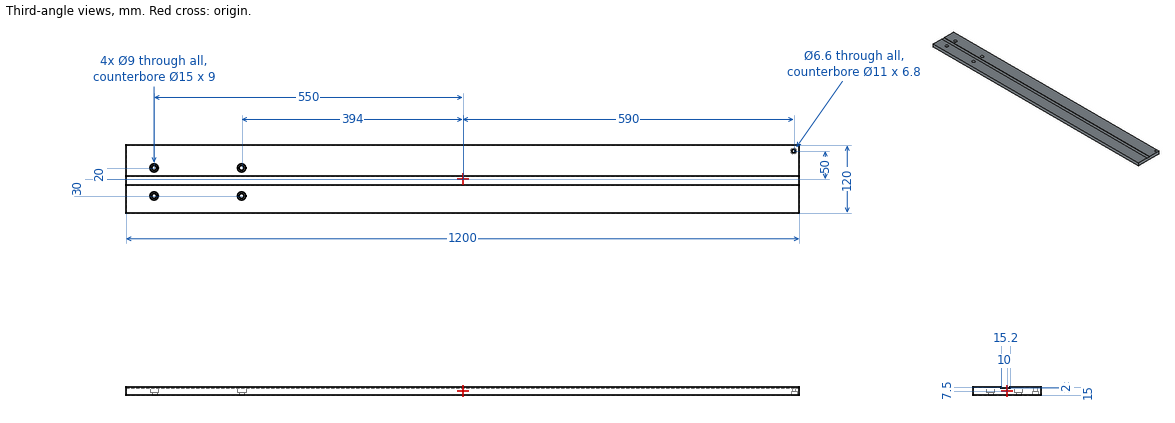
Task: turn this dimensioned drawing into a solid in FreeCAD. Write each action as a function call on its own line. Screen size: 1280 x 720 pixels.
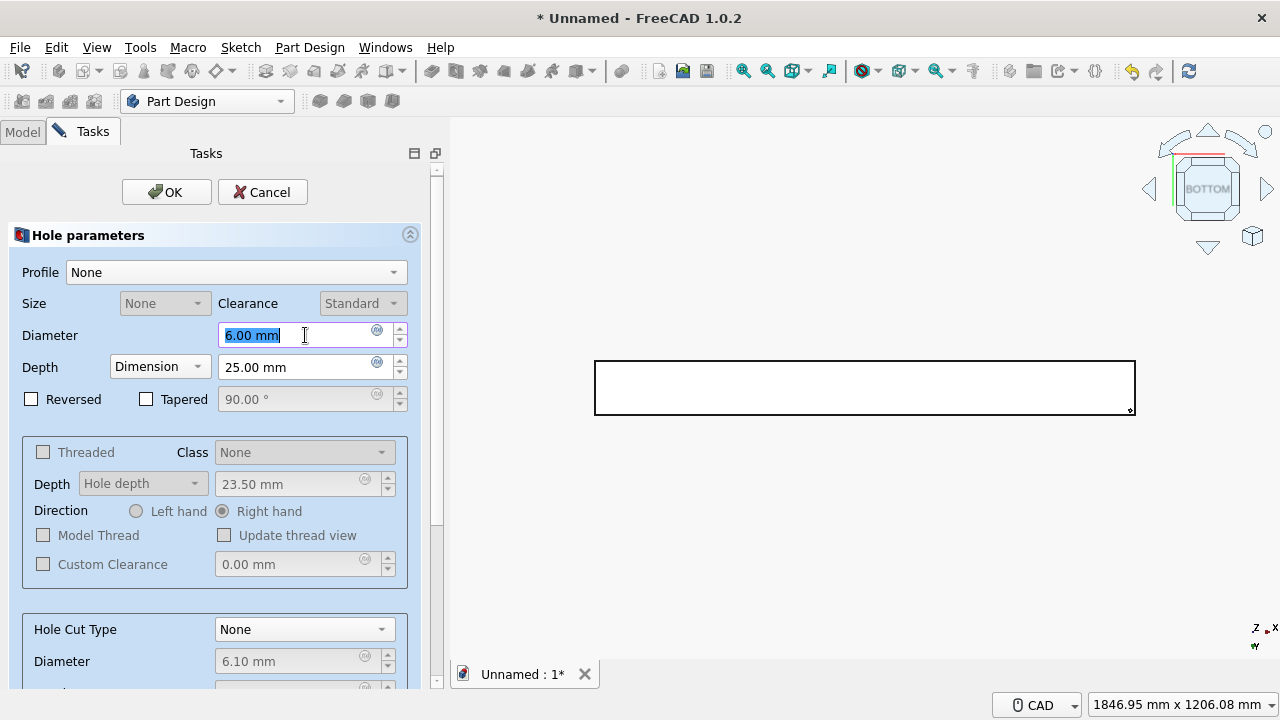
text(6.6)
key(Tab)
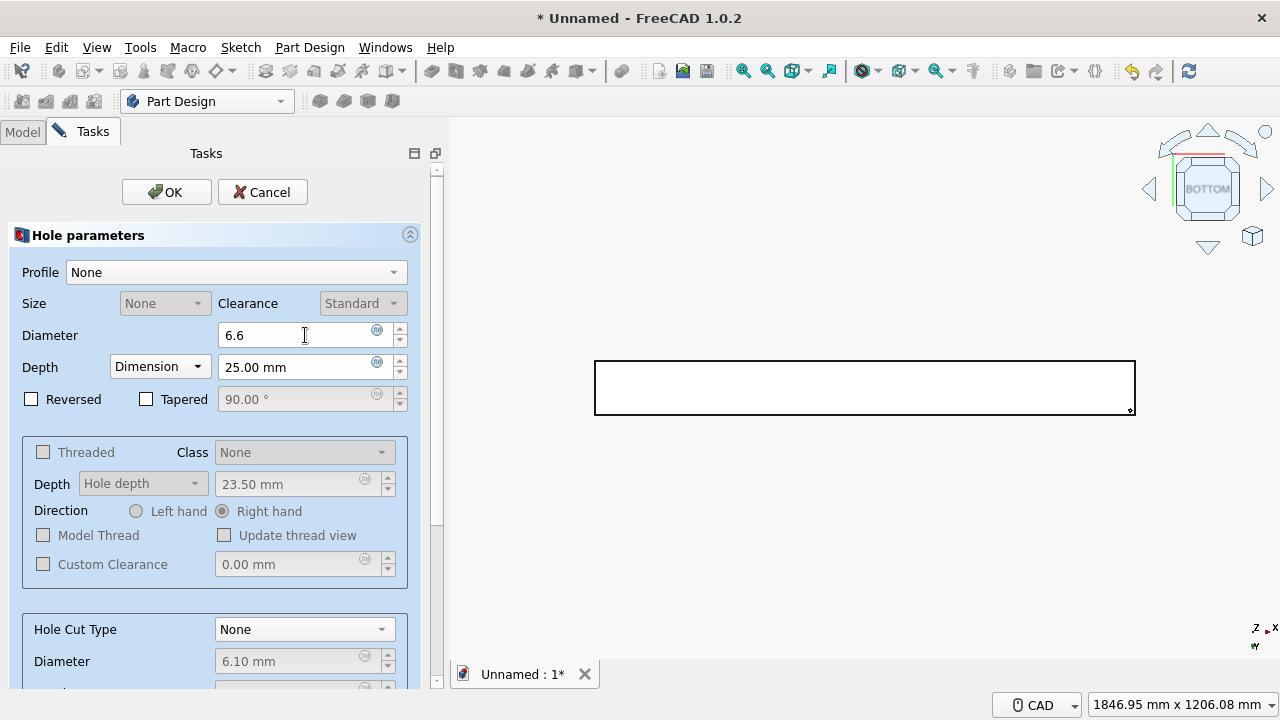
click(161, 366)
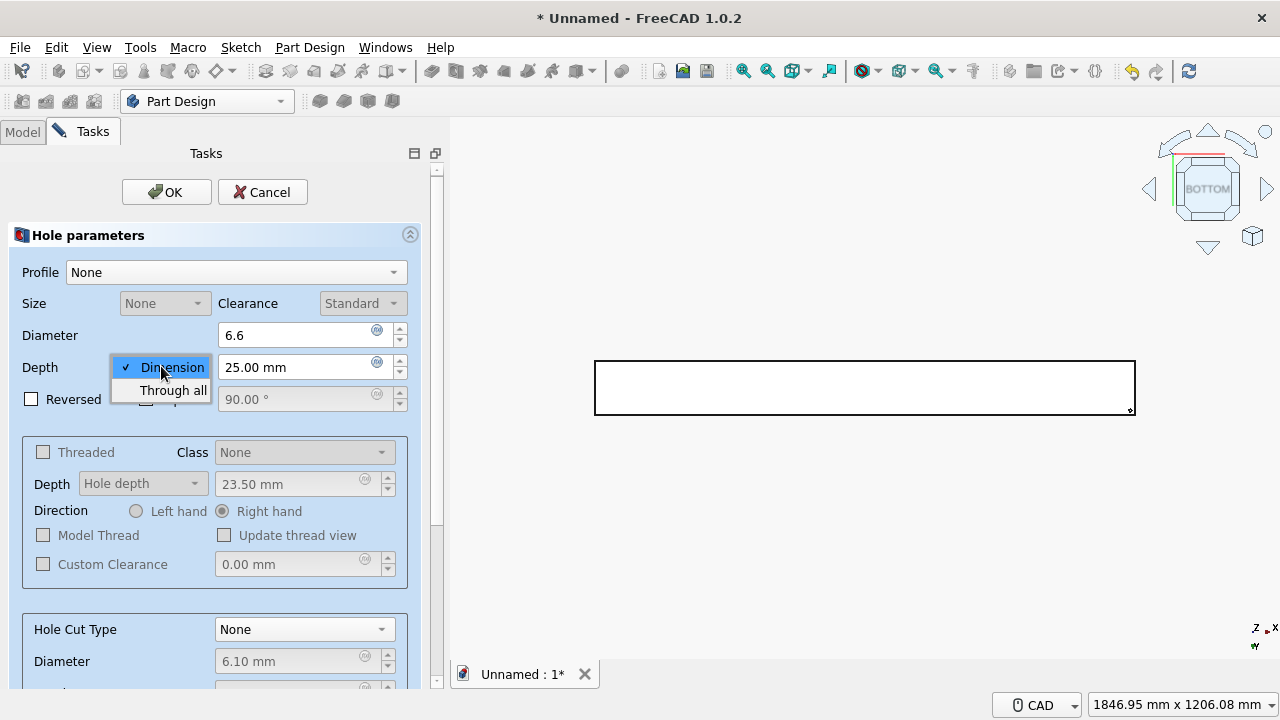
click(160, 390)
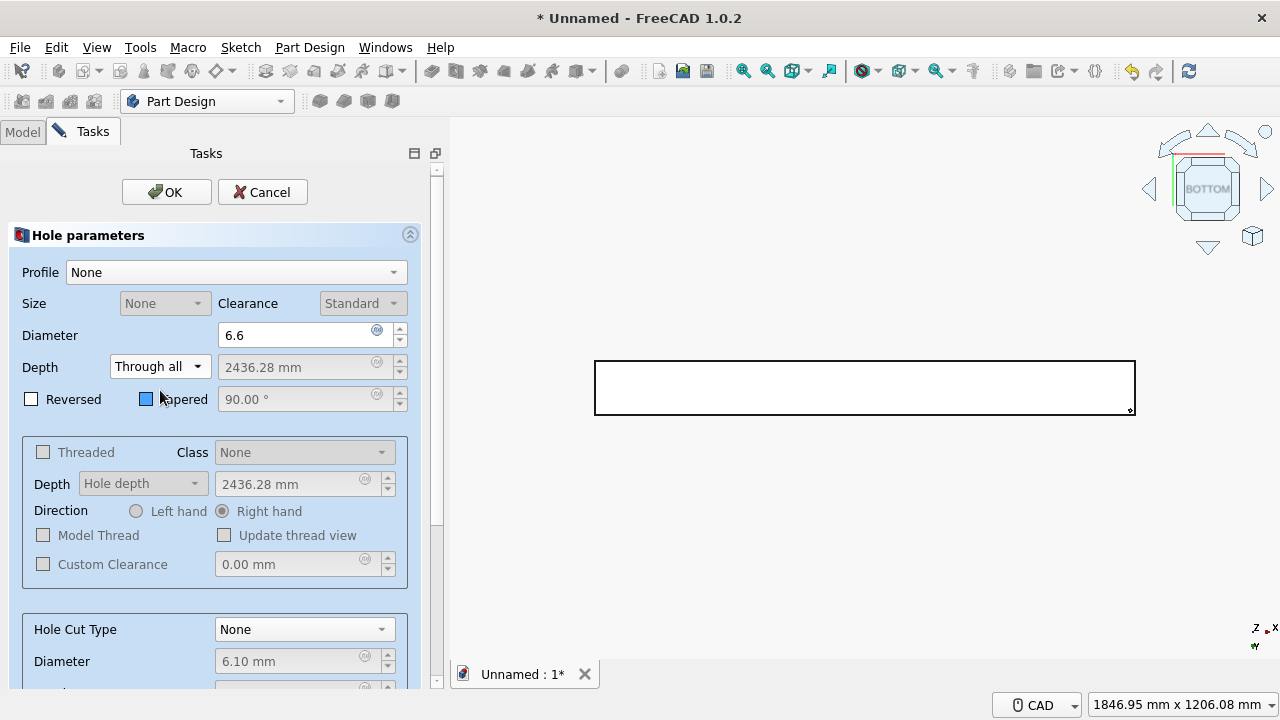
click(306, 630)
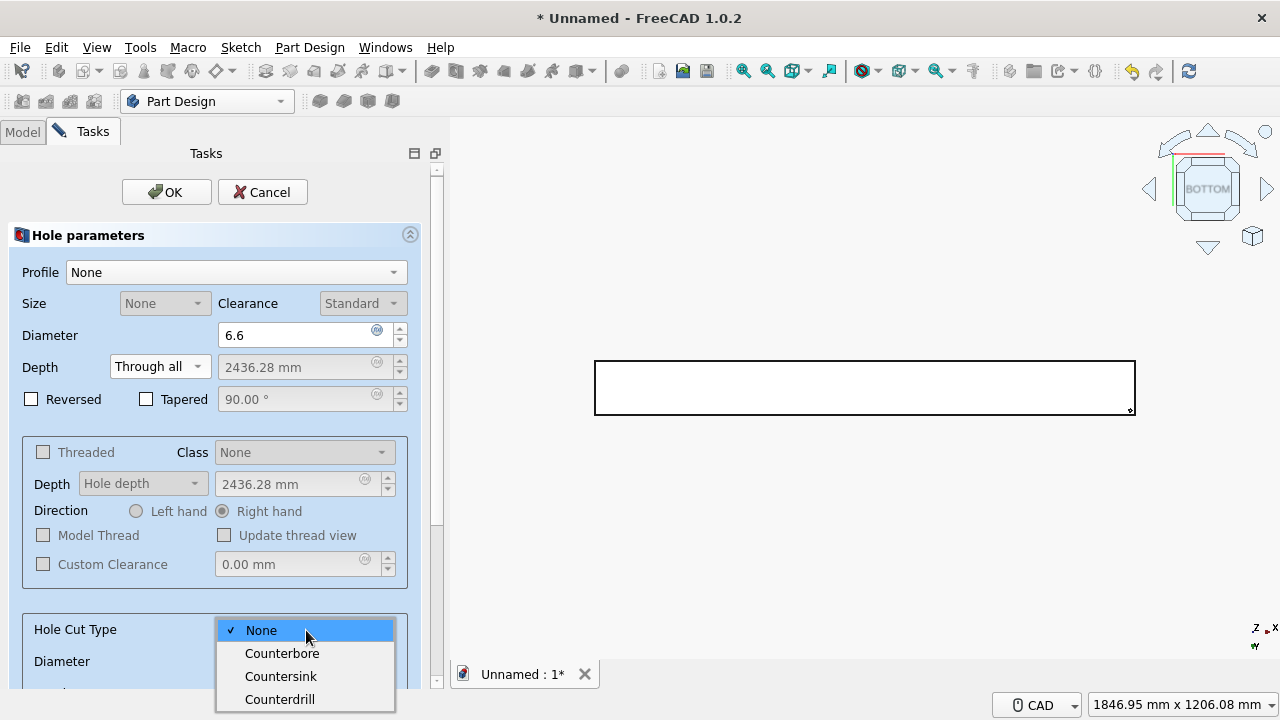
click(304, 654)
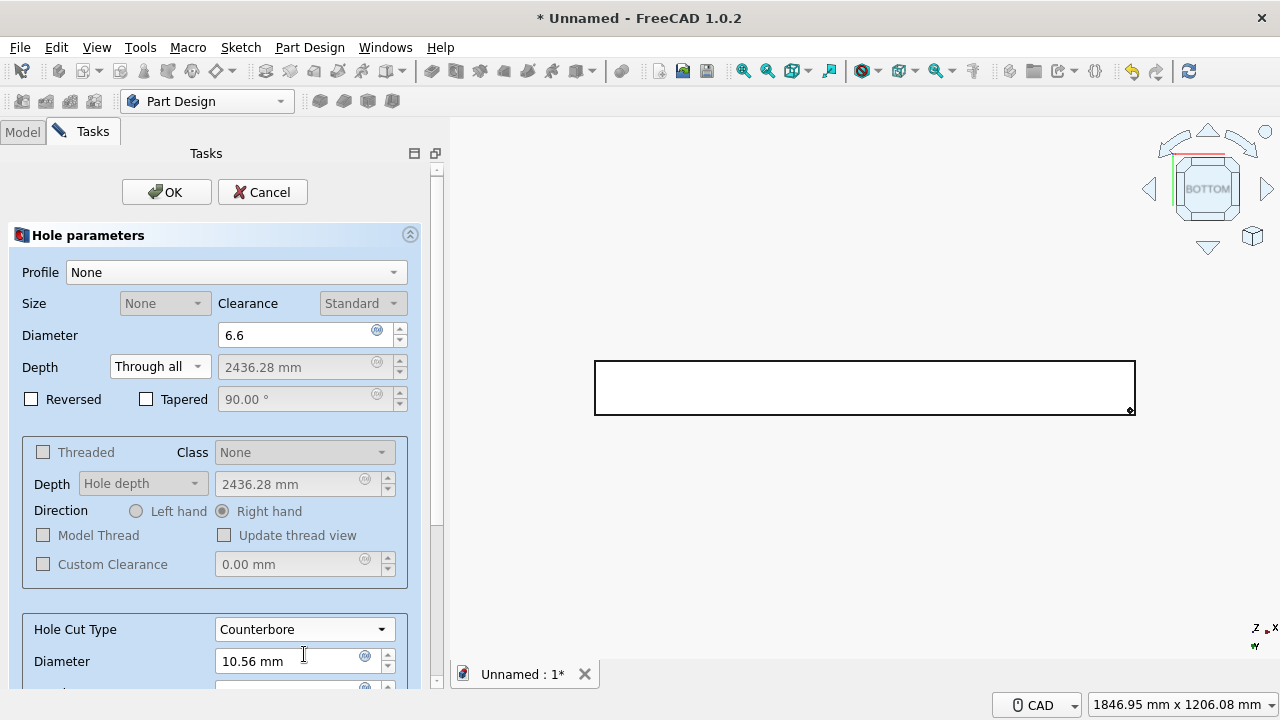
triple_click(298, 661)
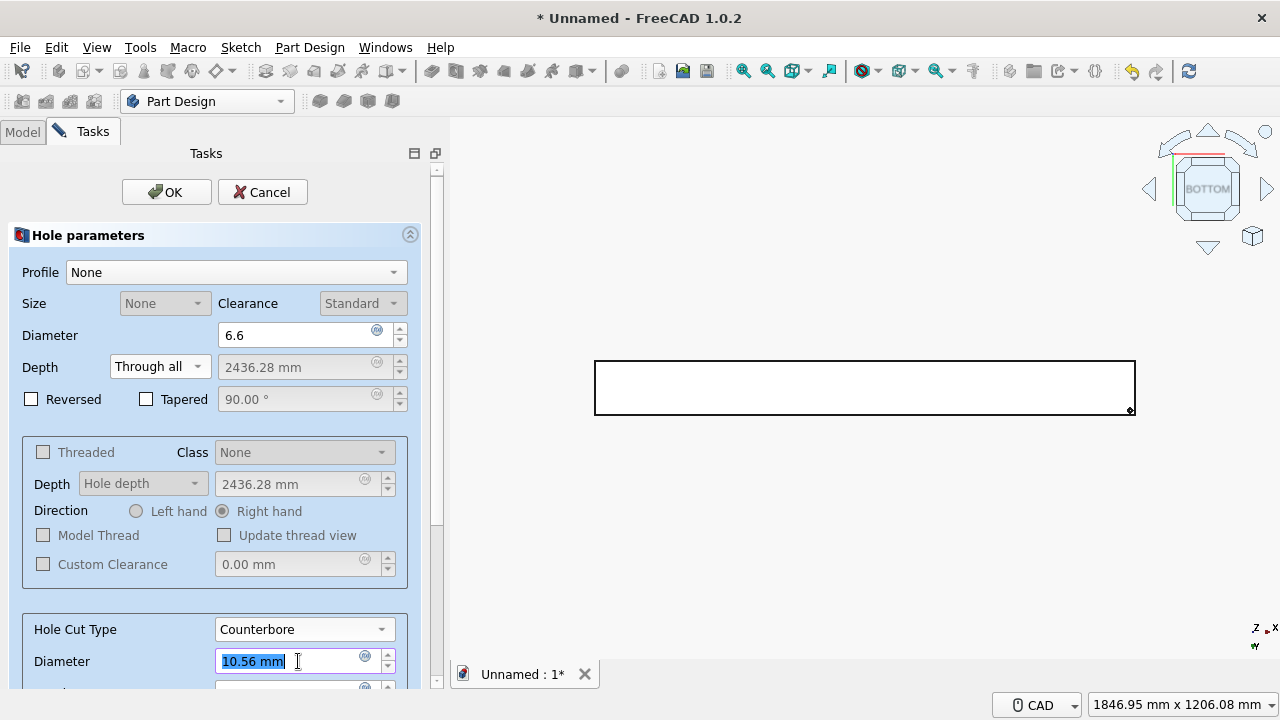
text(11)
key(Tab)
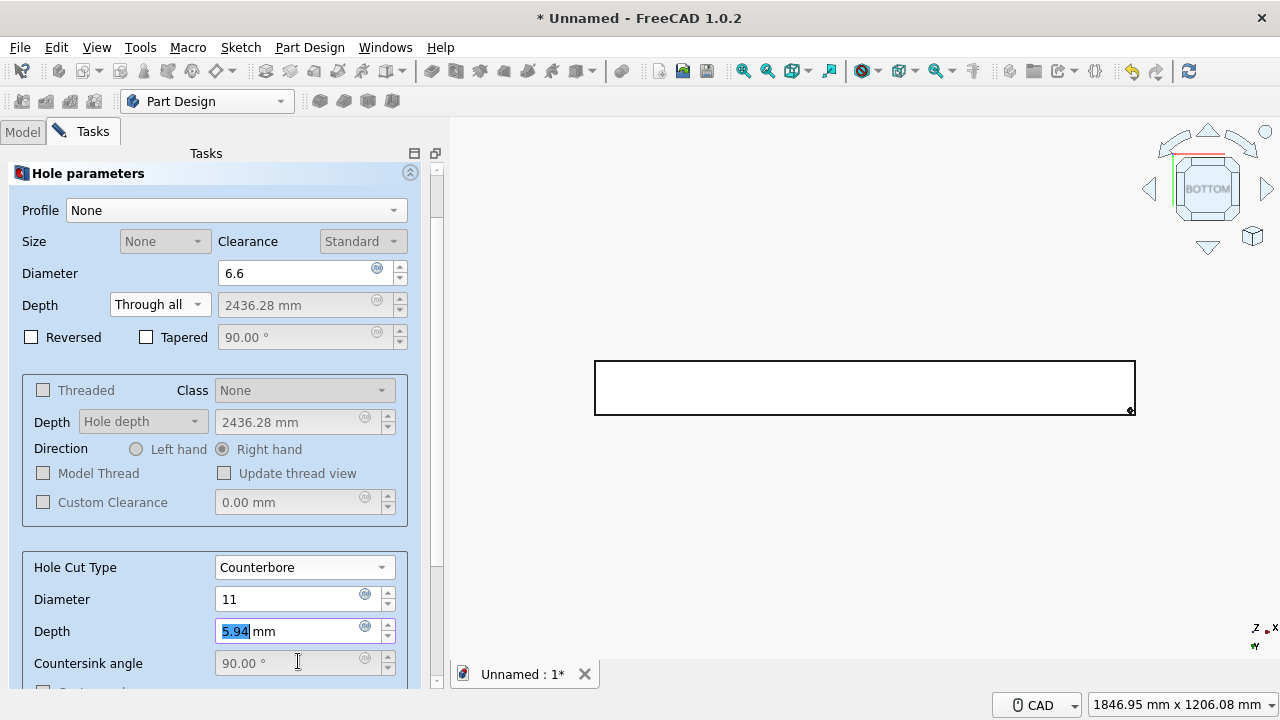
text(6.8)
key(Tab)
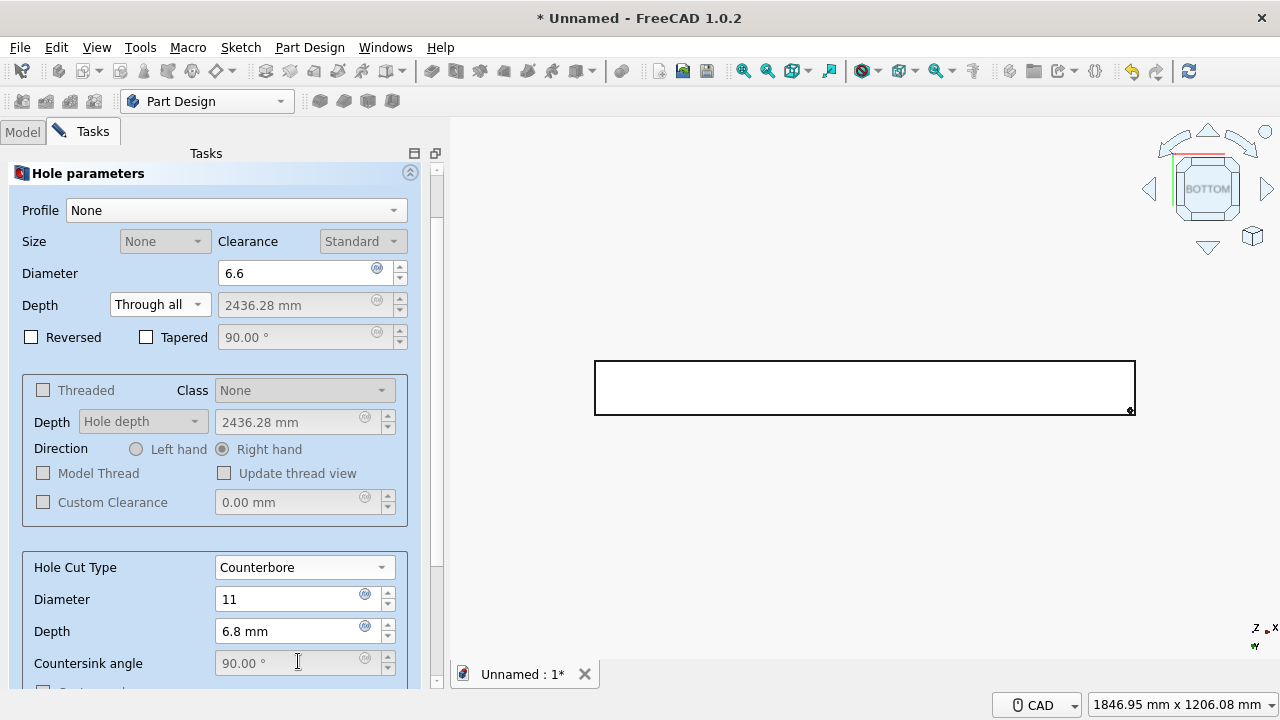
scroll(437, 426, up, 2)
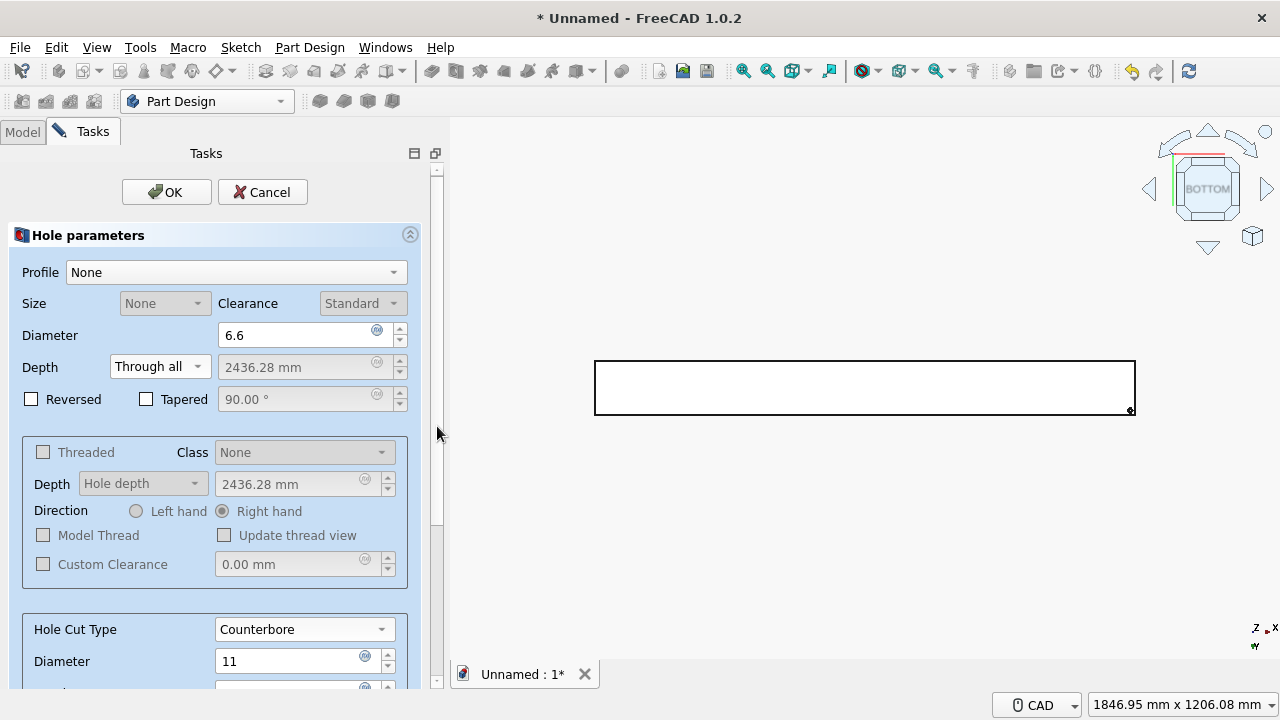
click(167, 192)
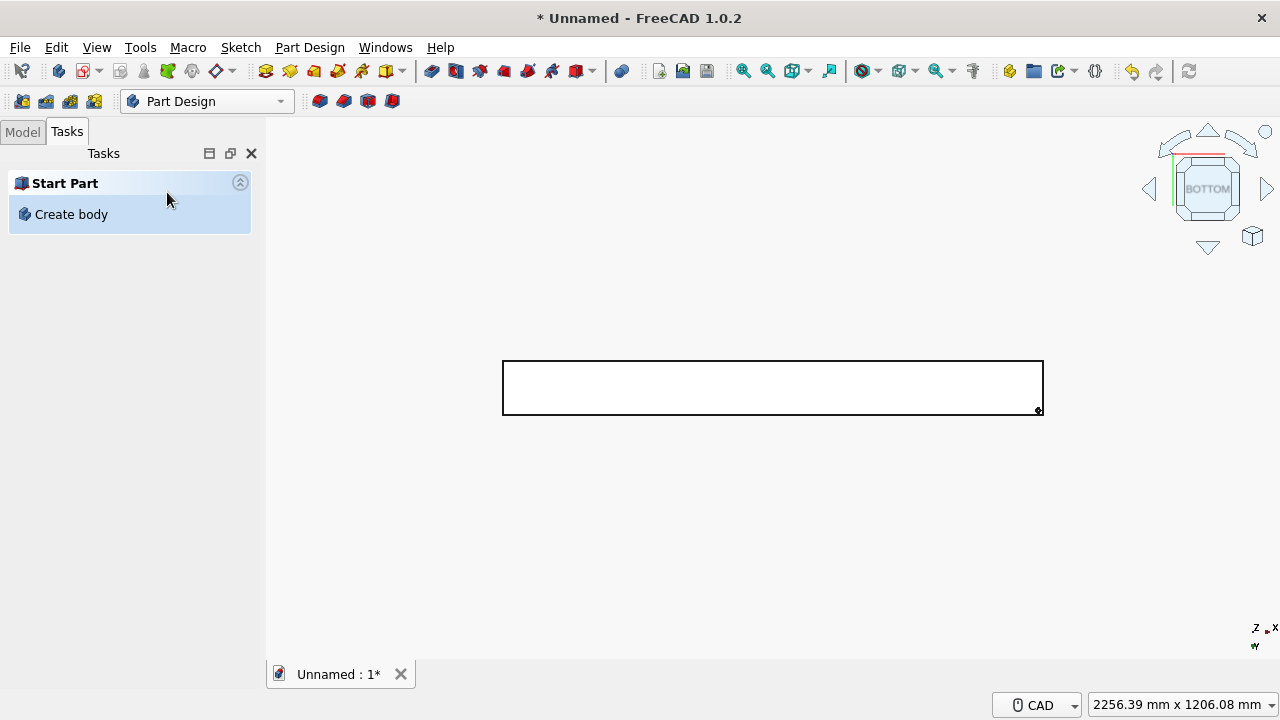
key(0)